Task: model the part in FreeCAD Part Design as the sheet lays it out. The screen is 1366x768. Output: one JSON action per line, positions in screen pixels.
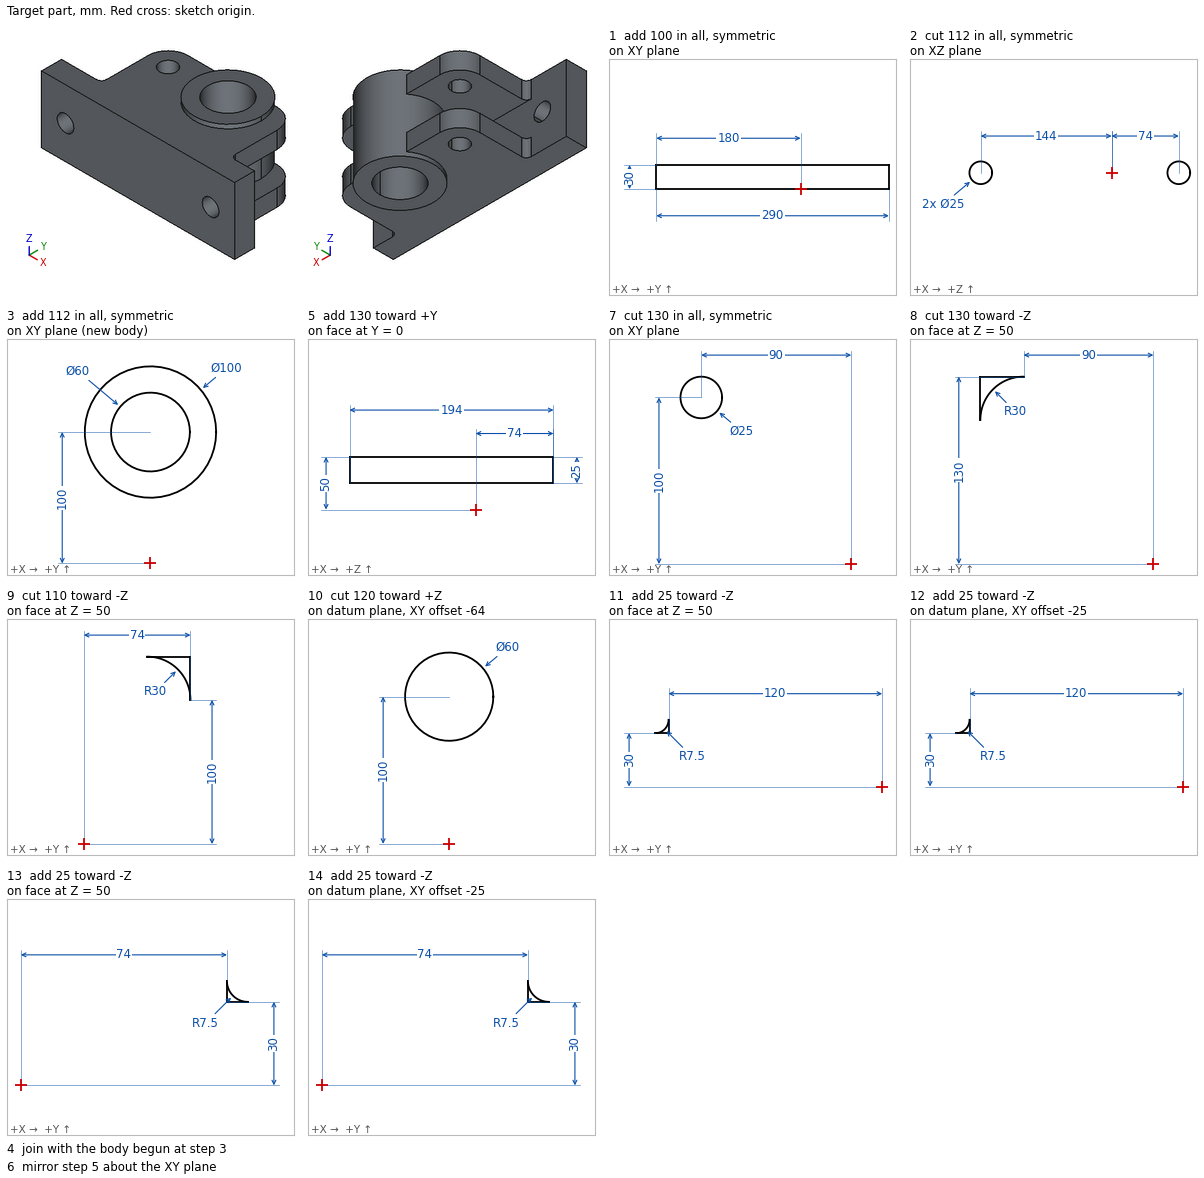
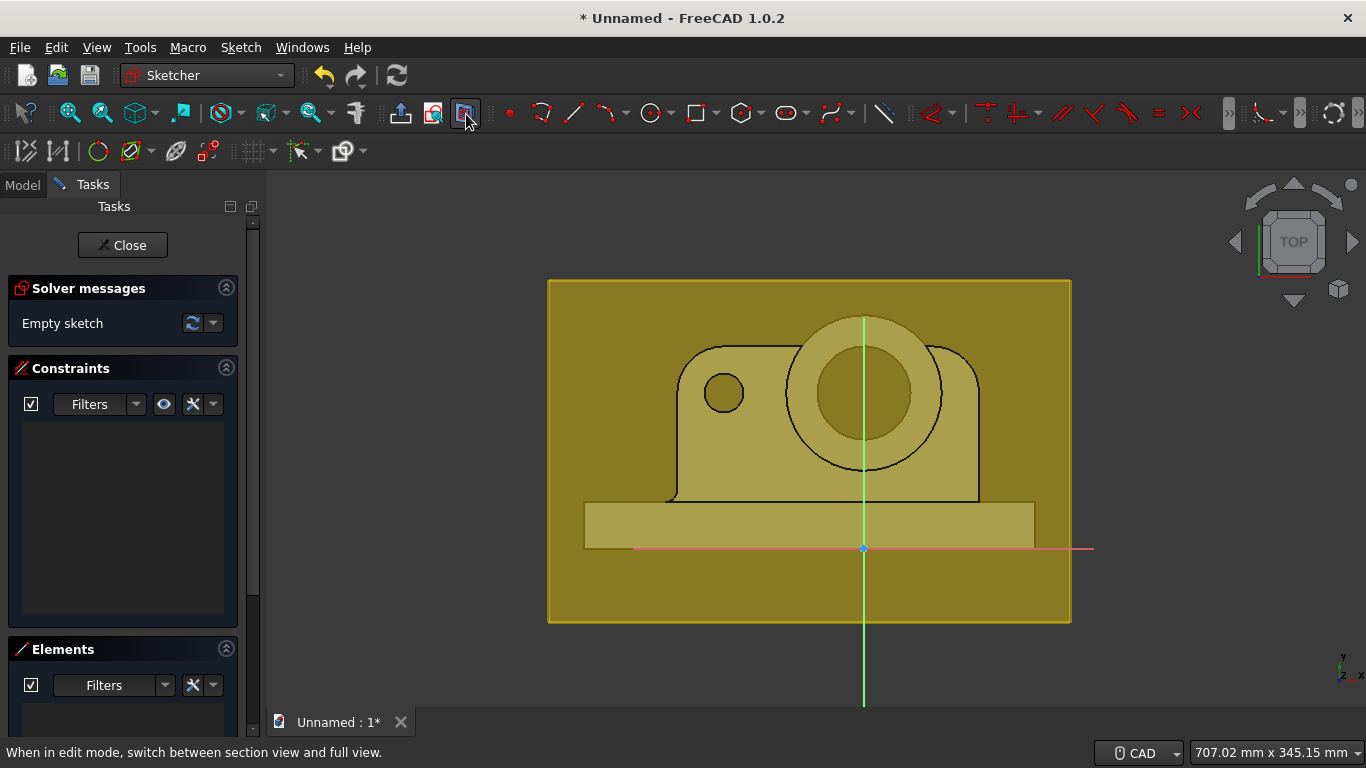
{"action": "scroll", "coordinate": [997, 499], "scroll_direction": "up", "scroll_amount": 15}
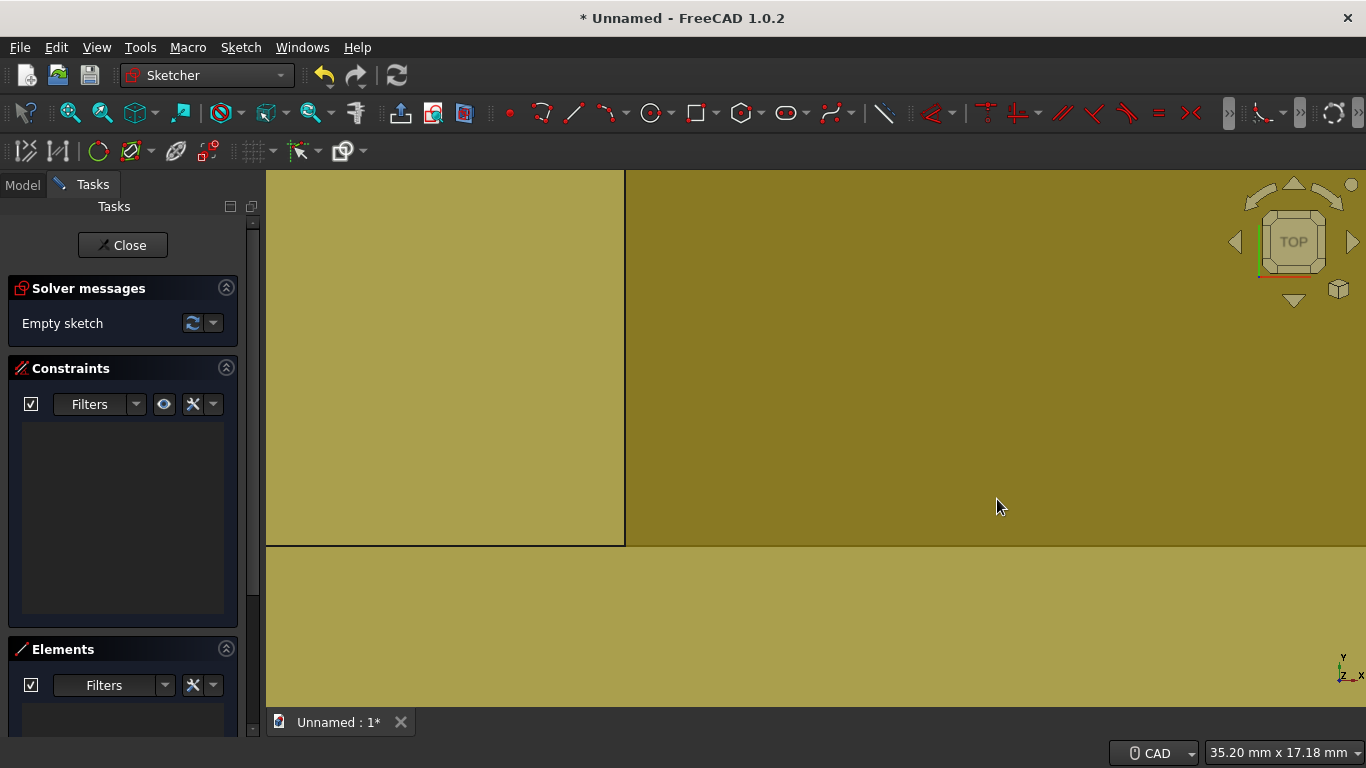
{"action": "scroll", "coordinate": [731, 408], "scroll_direction": "up", "scroll_amount": 2}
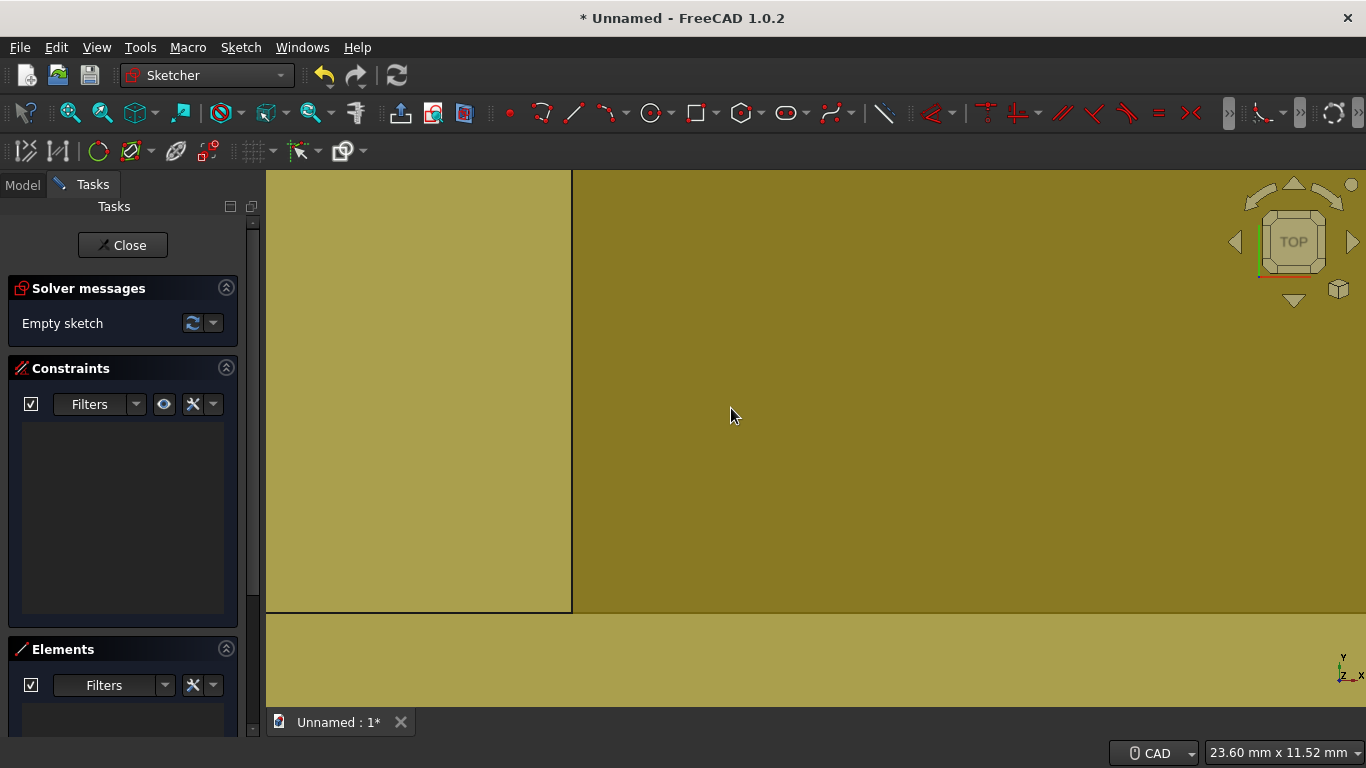
{"action": "left_click", "coordinate": [542, 114]}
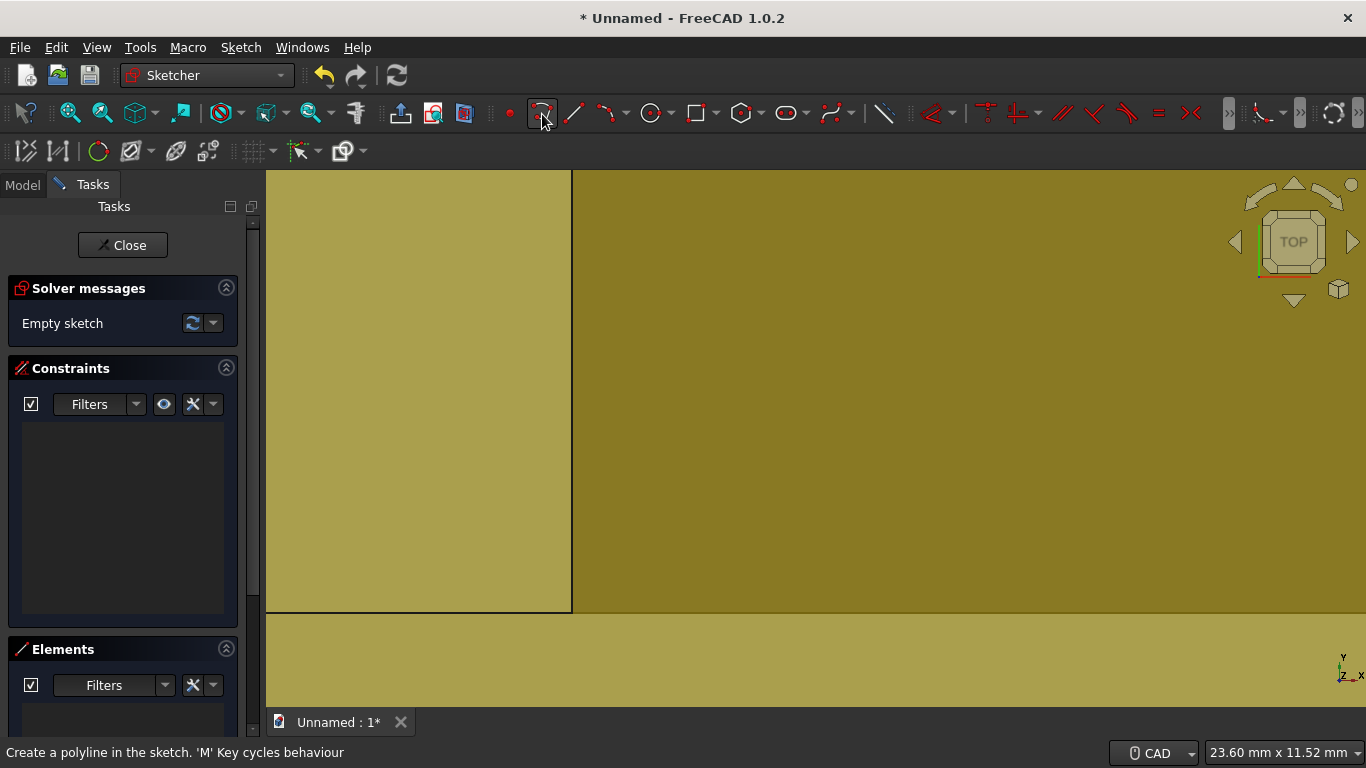
{"action": "left_click", "coordinate": [572, 263]}
{"action": "left_click", "coordinate": [572, 613]}
{"action": "left_click", "coordinate": [922, 613]}
{"action": "right_click", "coordinate": [922, 613]}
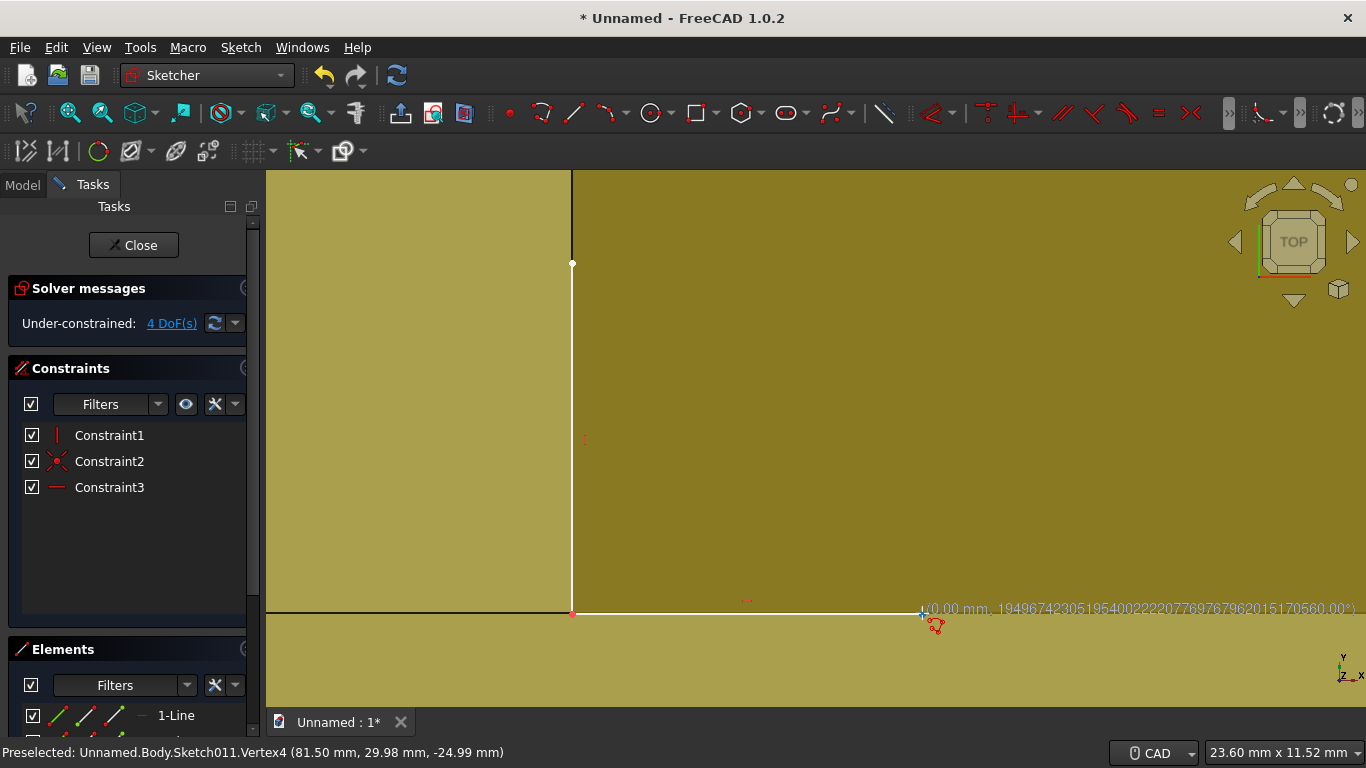
{"action": "left_click", "coordinate": [606, 114]}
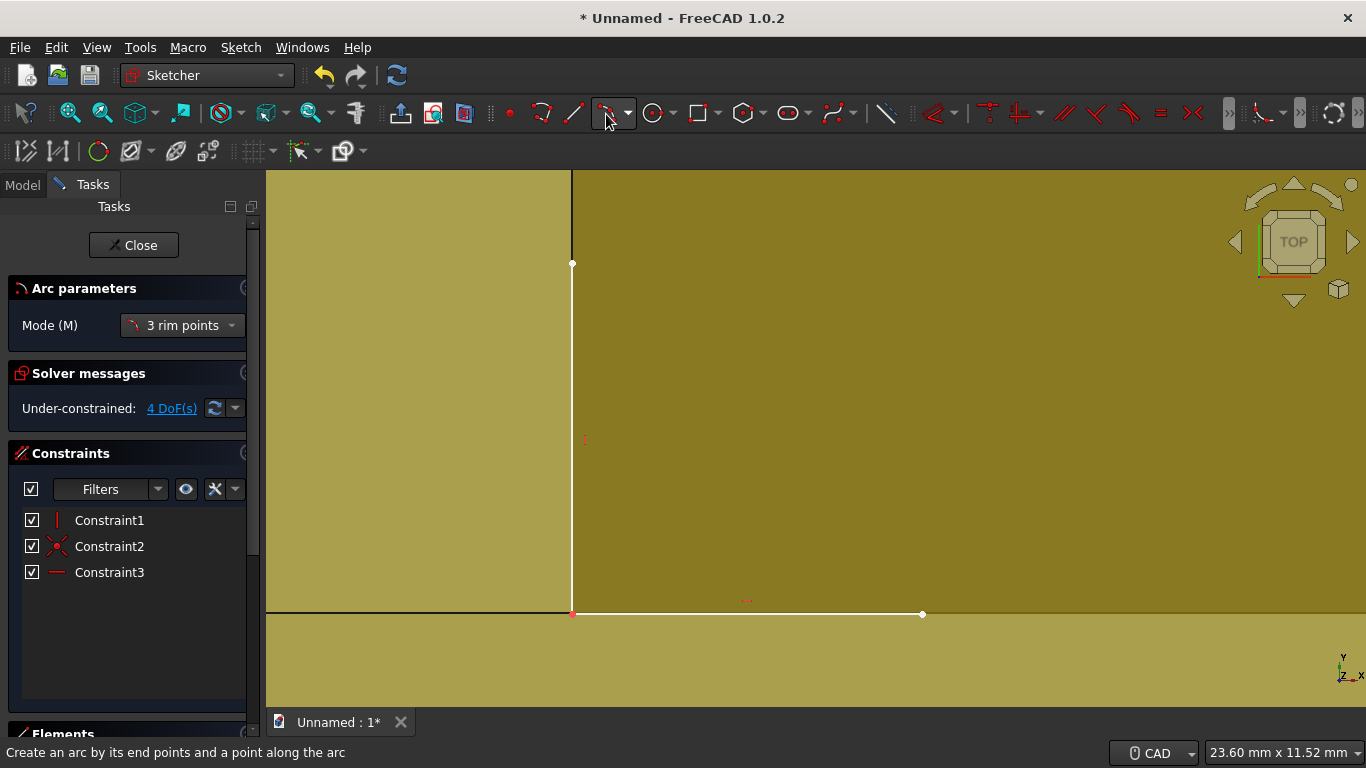
{"action": "left_click", "coordinate": [922, 614]}
{"action": "left_click", "coordinate": [572, 264]}
{"action": "left_click", "coordinate": [675, 511]}
{"action": "key", "text": "Escape"}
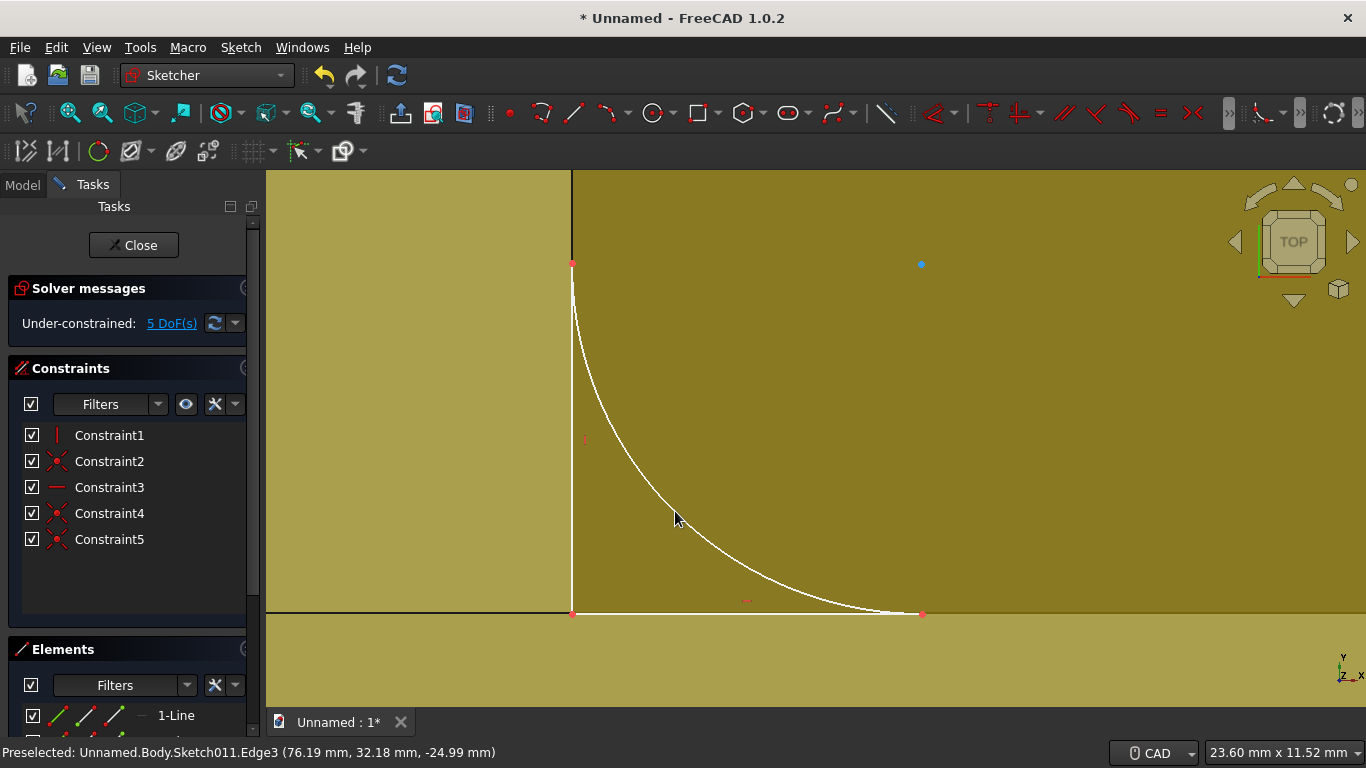
{"action": "left_click", "coordinate": [572, 369]}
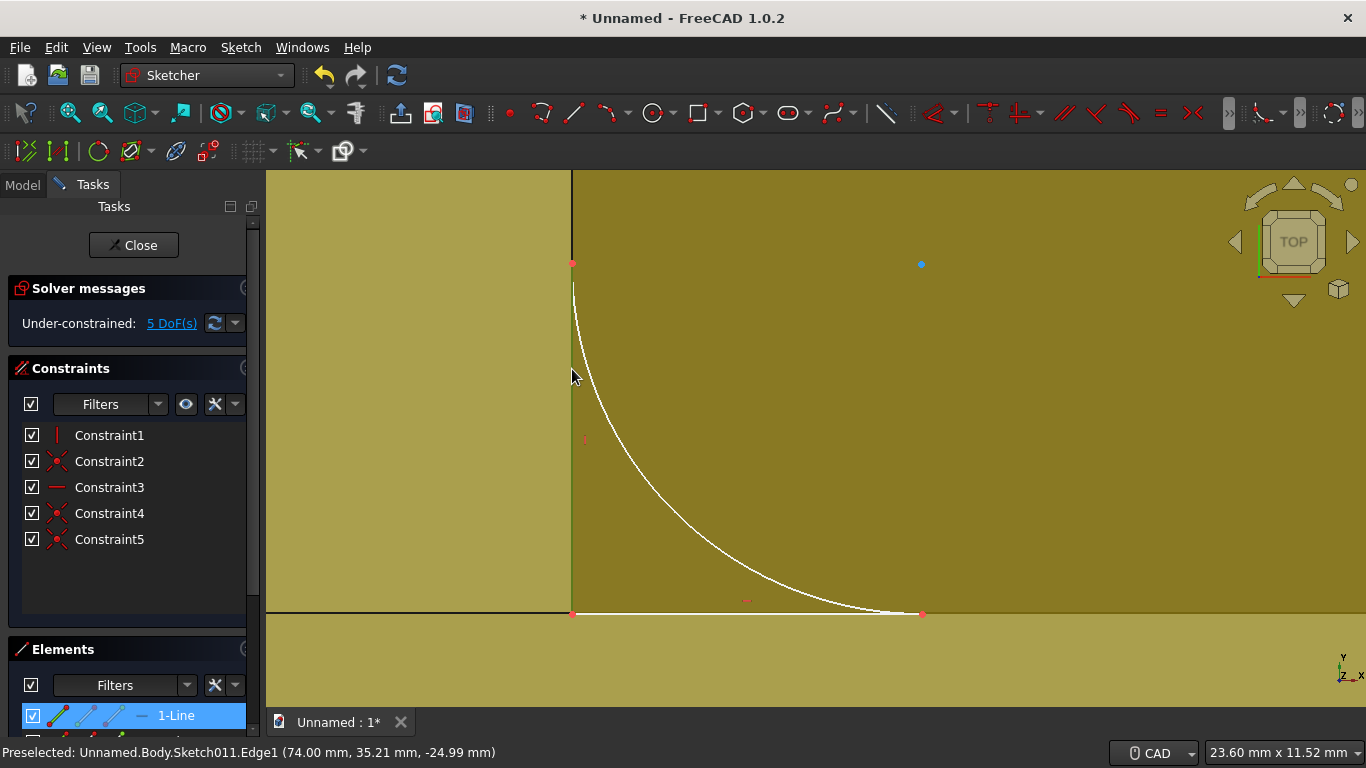
{"action": "left_click", "coordinate": [610, 423]}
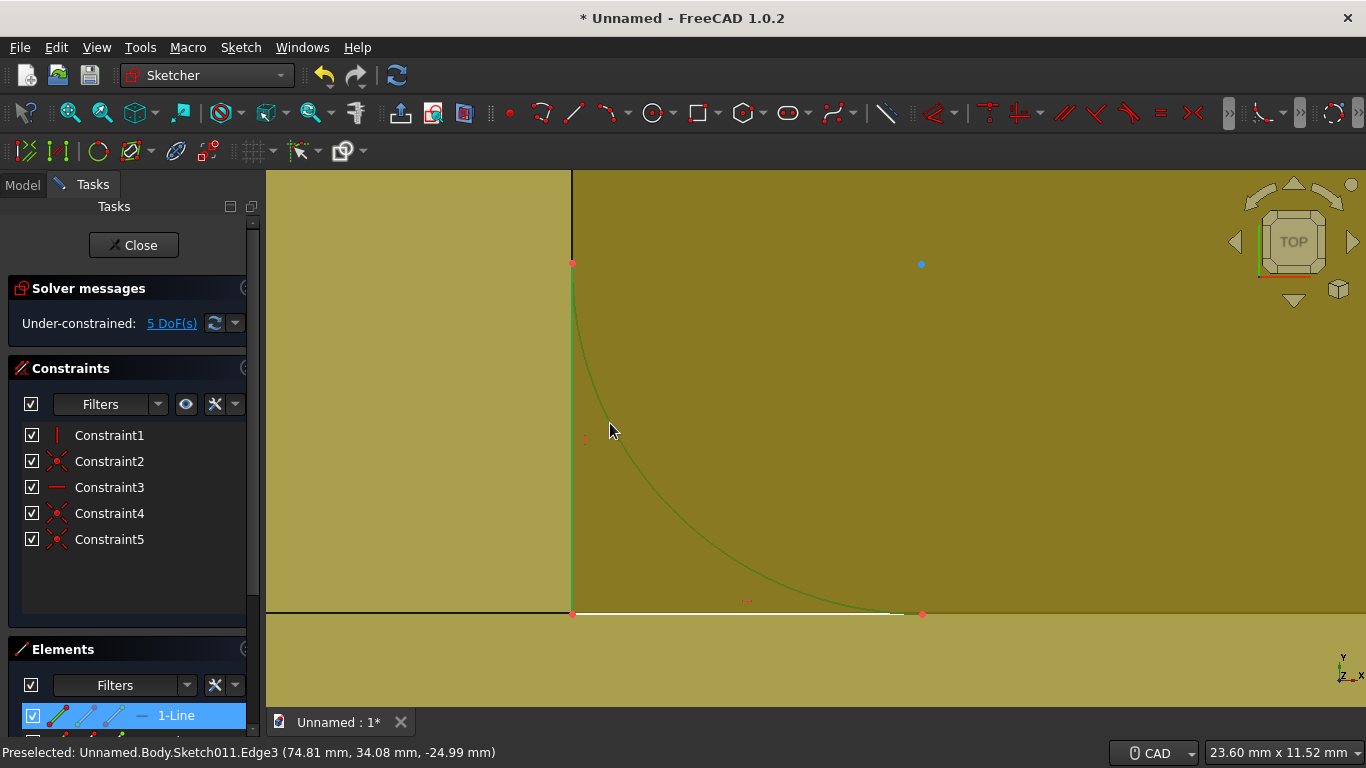
{"action": "left_click", "coordinate": [1130, 114]}